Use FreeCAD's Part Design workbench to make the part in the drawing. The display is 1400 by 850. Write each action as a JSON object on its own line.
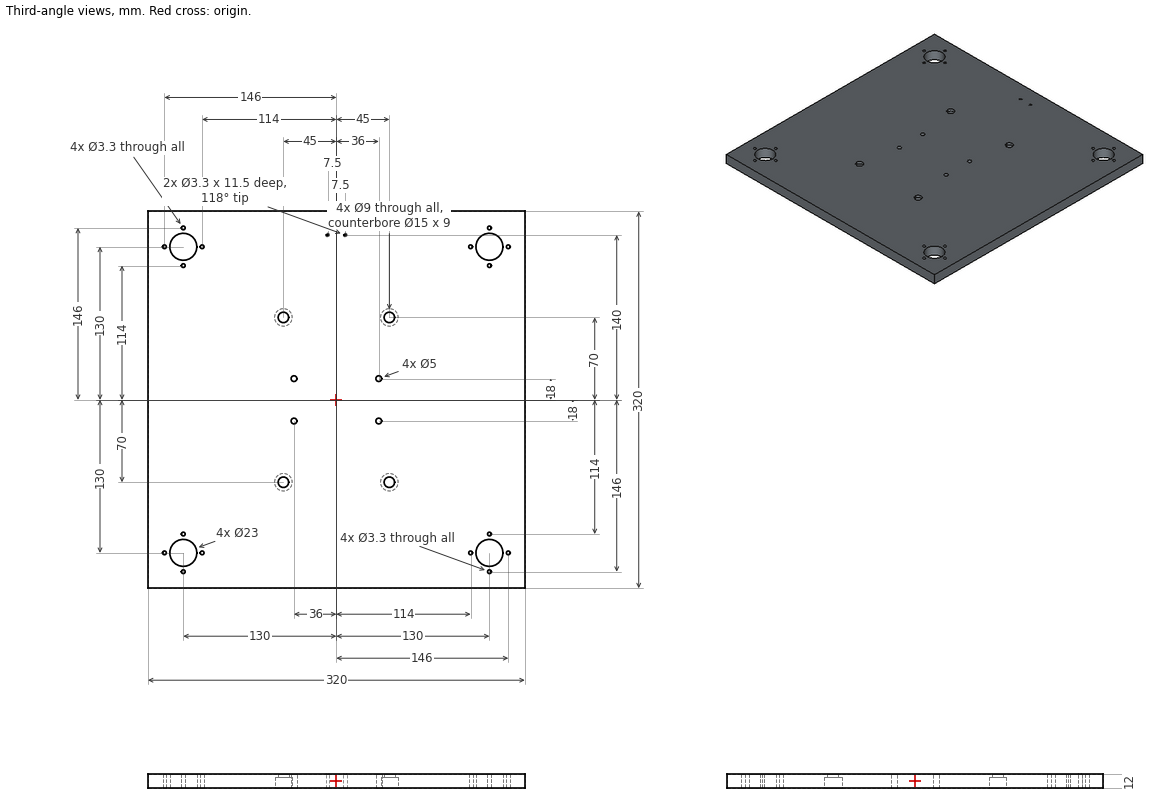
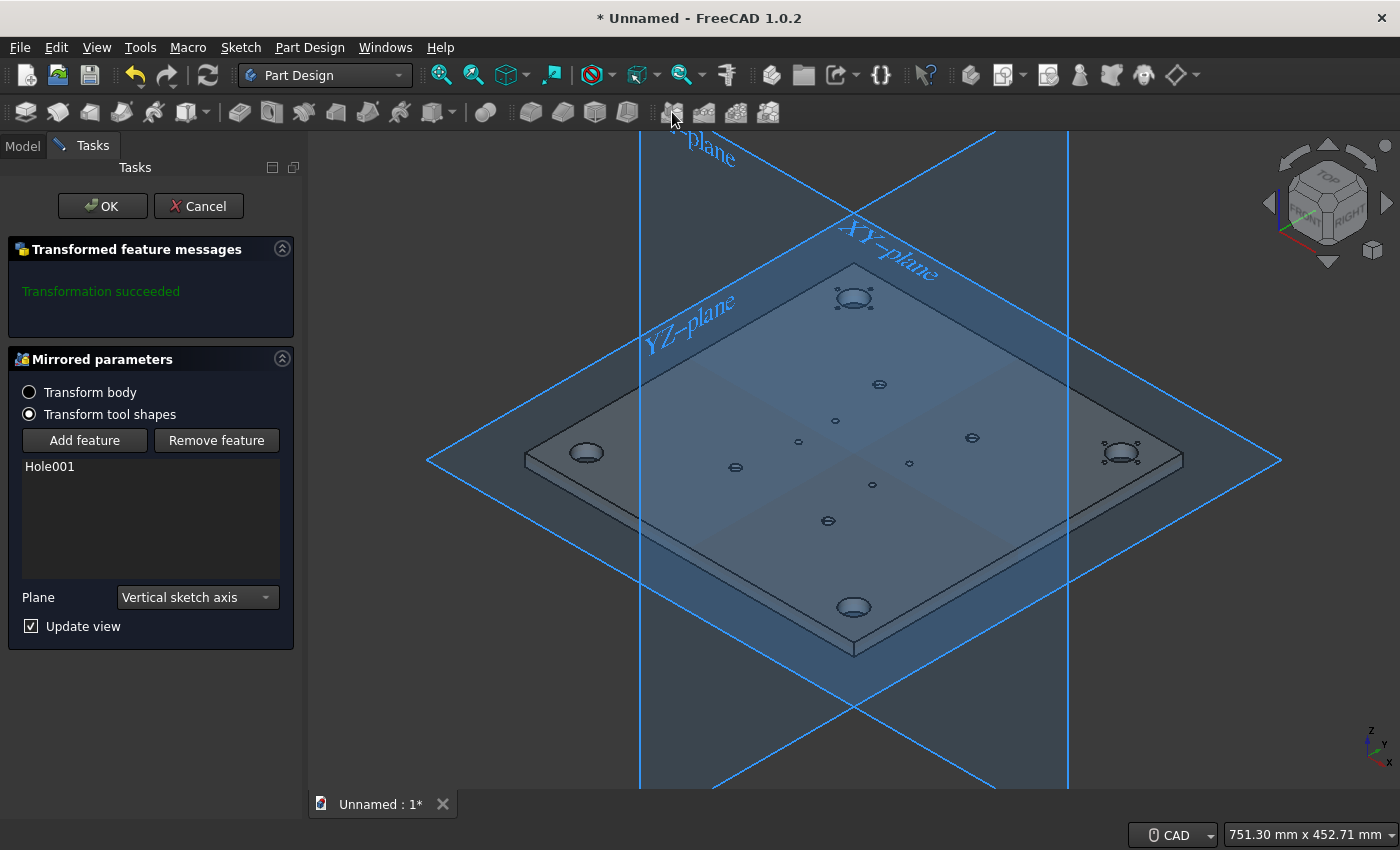
{"action": "left_click", "coordinate": [198, 598]}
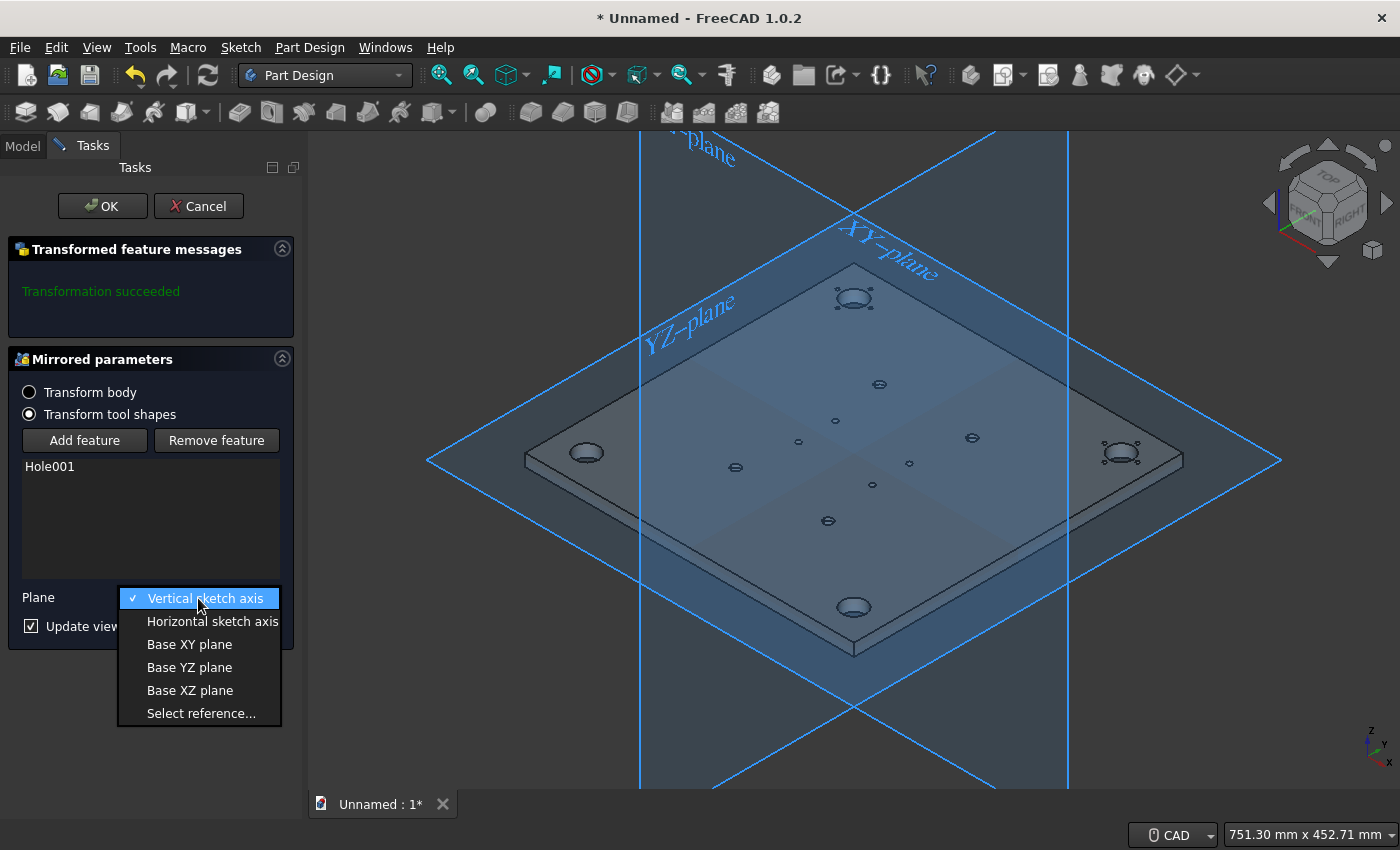
{"action": "left_click", "coordinate": [198, 690]}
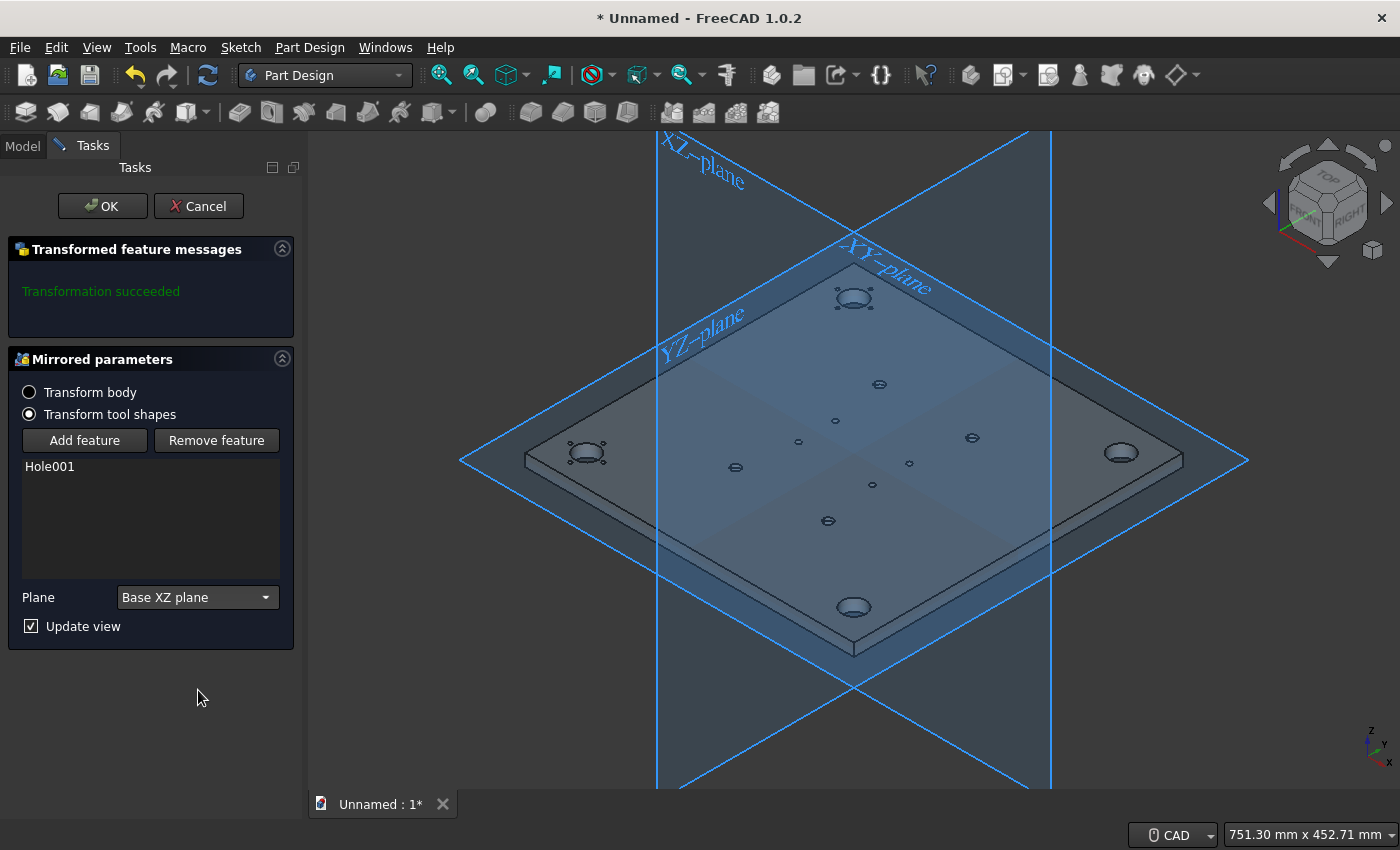
{"action": "left_click", "coordinate": [103, 206]}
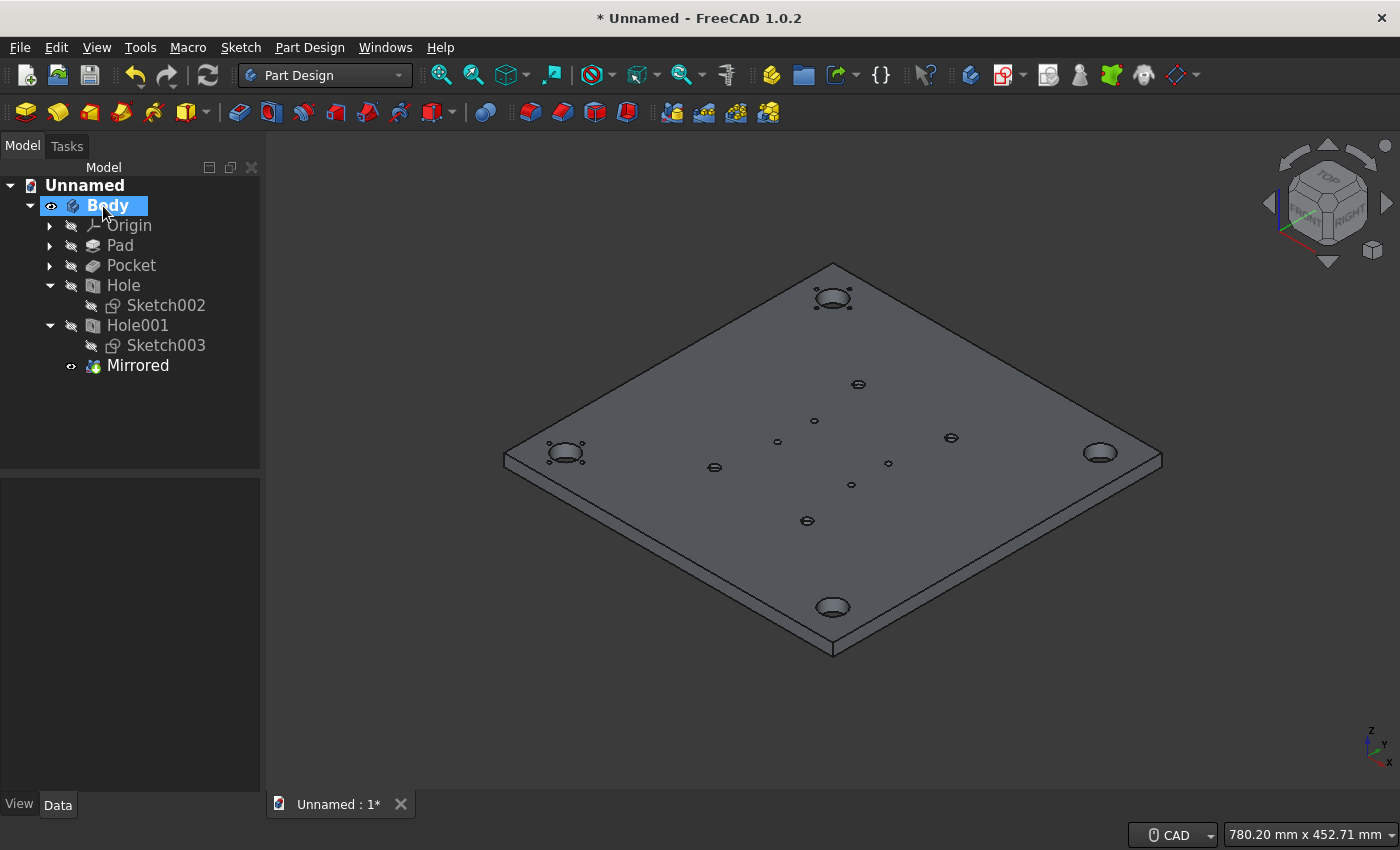
{"action": "left_click", "coordinate": [116, 326]}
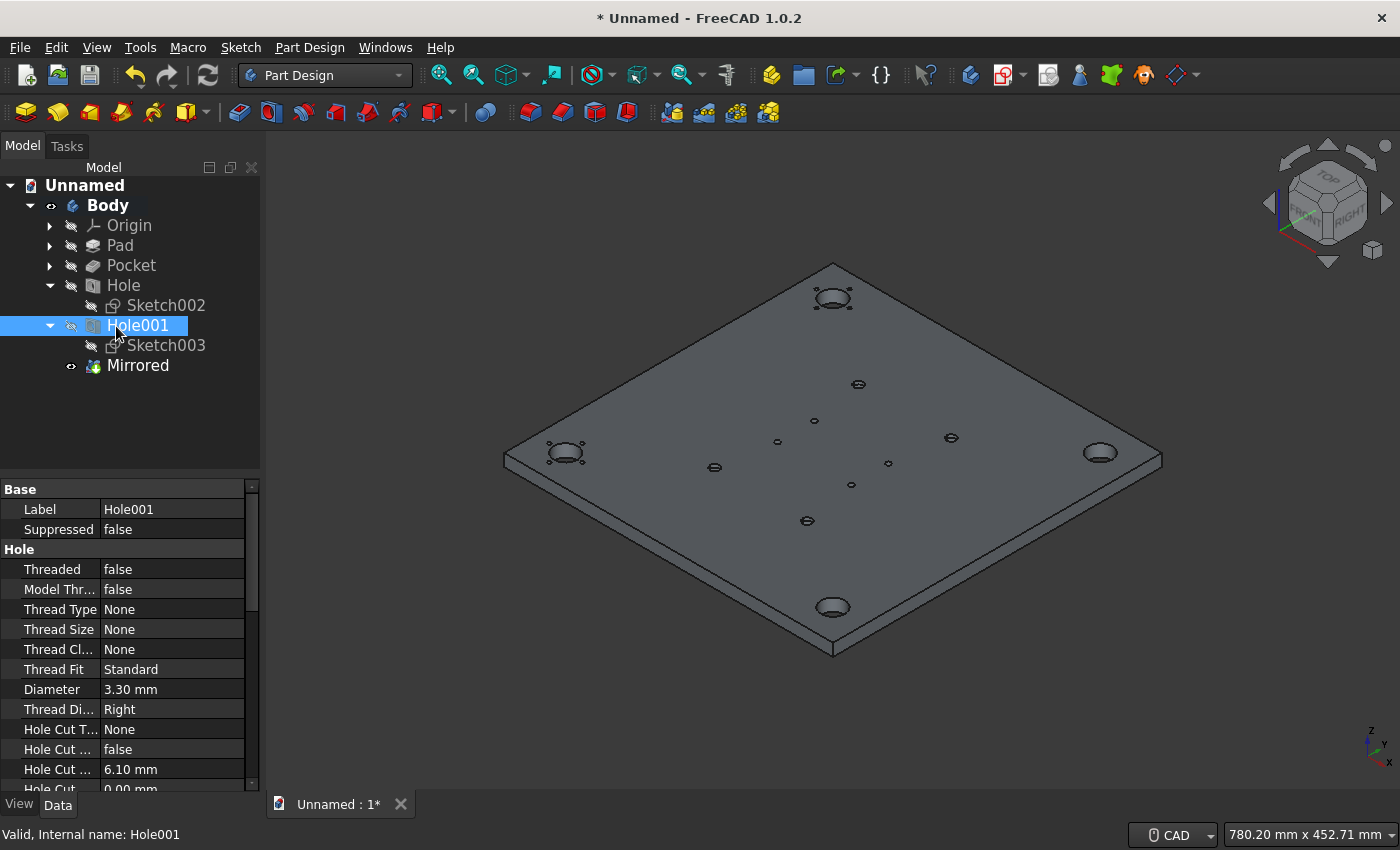
{"action": "left_click", "coordinate": [672, 112]}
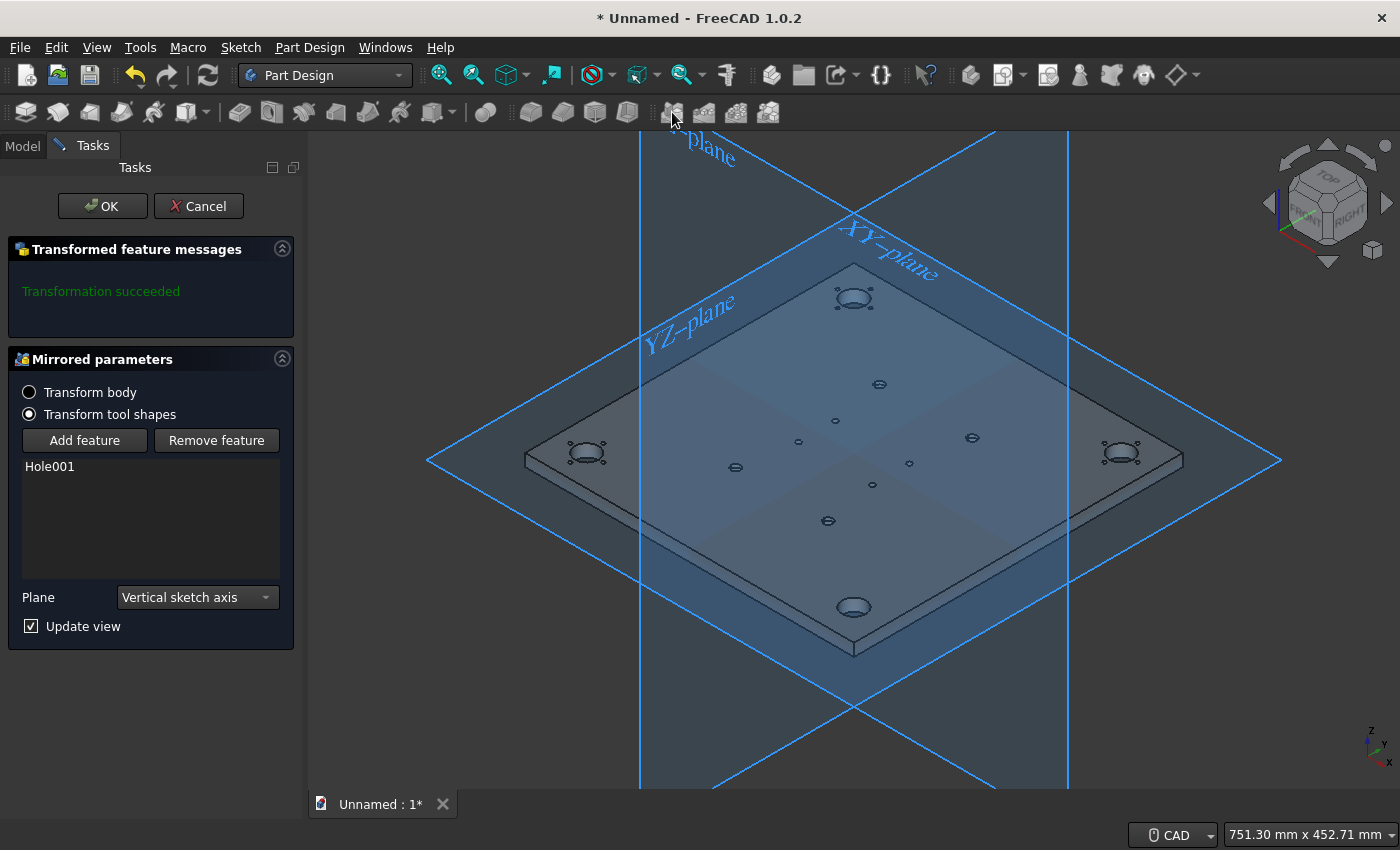
{"action": "left_click", "coordinate": [198, 598]}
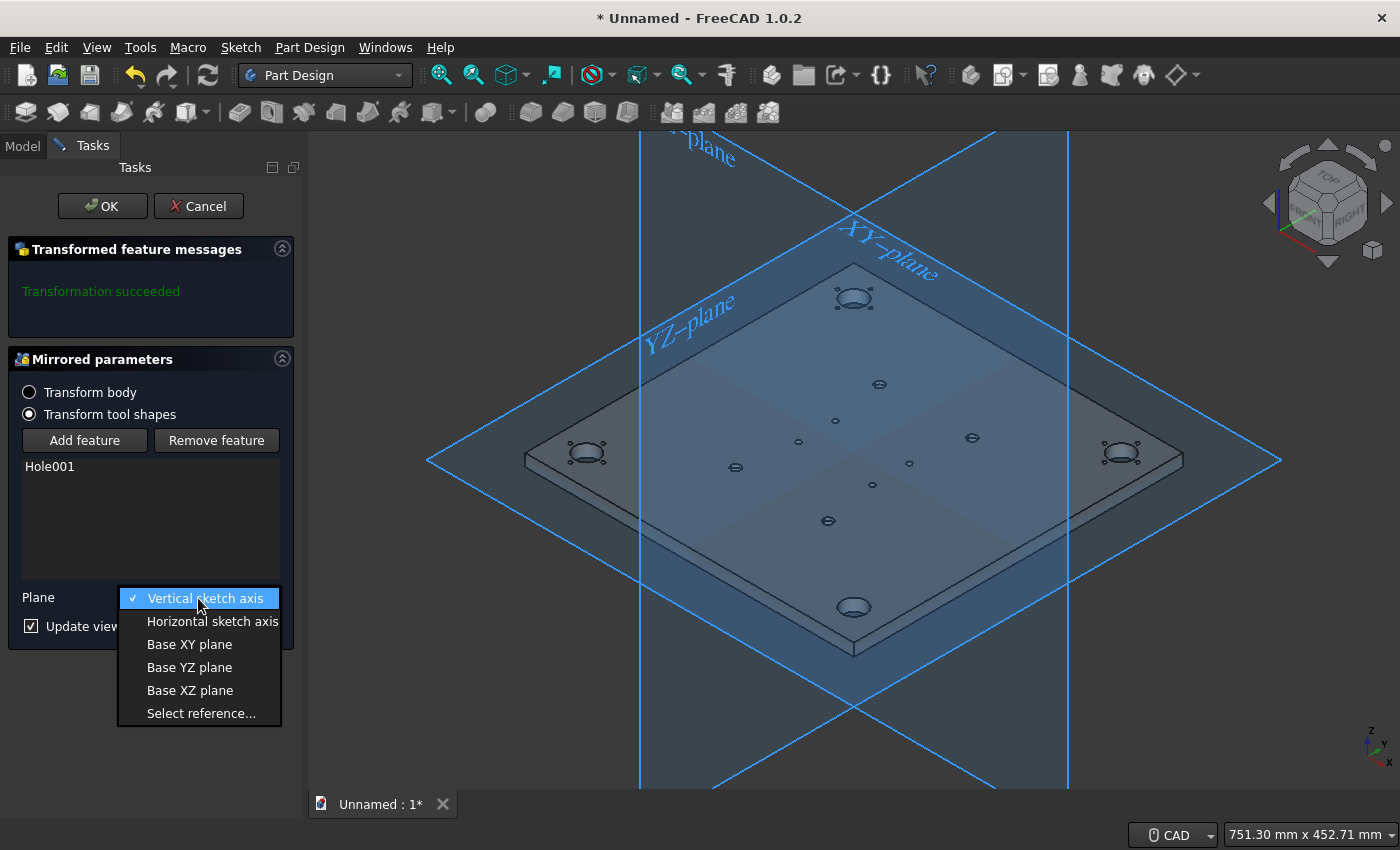
{"action": "left_click", "coordinate": [198, 668]}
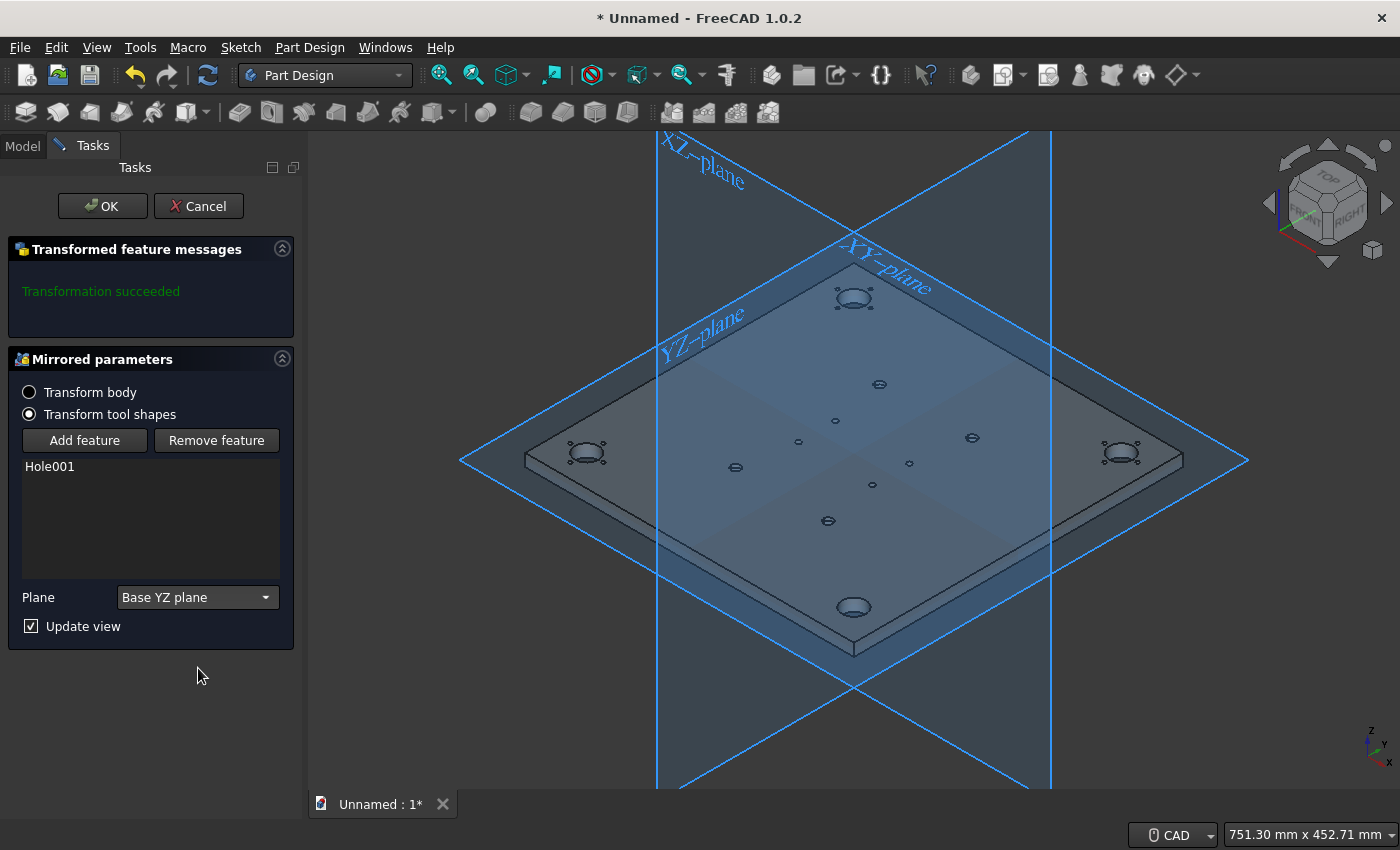
{"action": "left_click", "coordinate": [103, 206]}